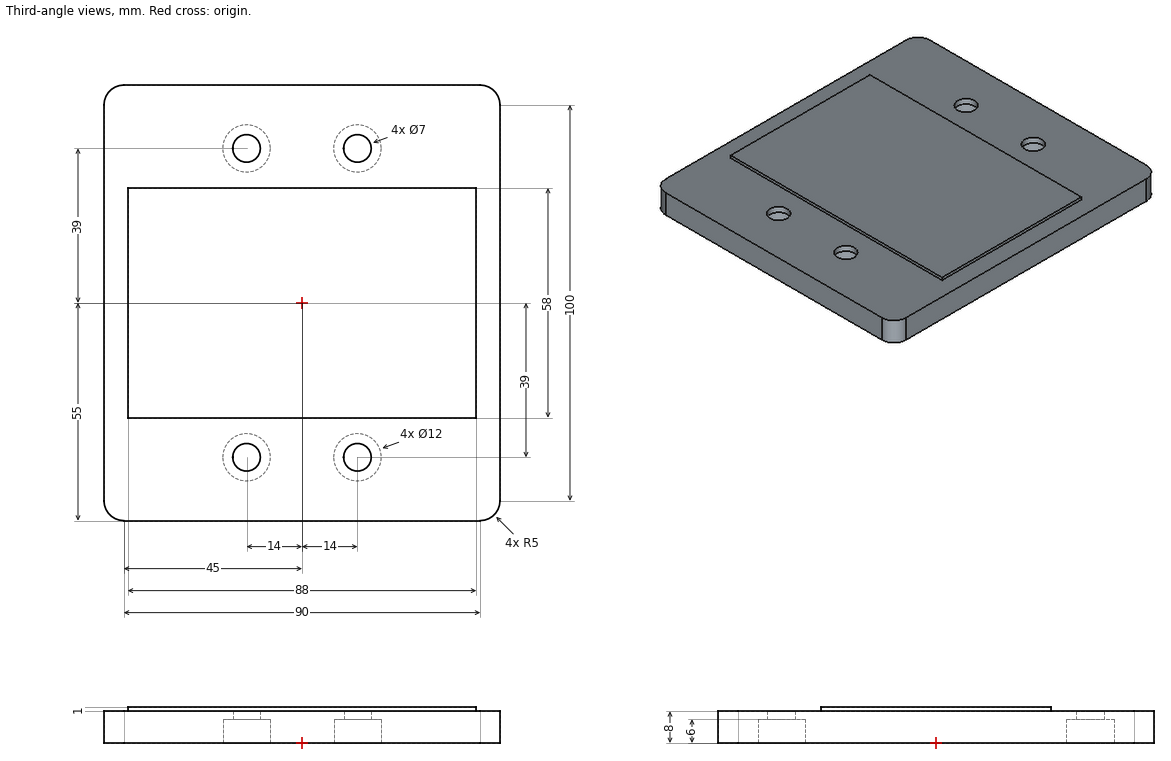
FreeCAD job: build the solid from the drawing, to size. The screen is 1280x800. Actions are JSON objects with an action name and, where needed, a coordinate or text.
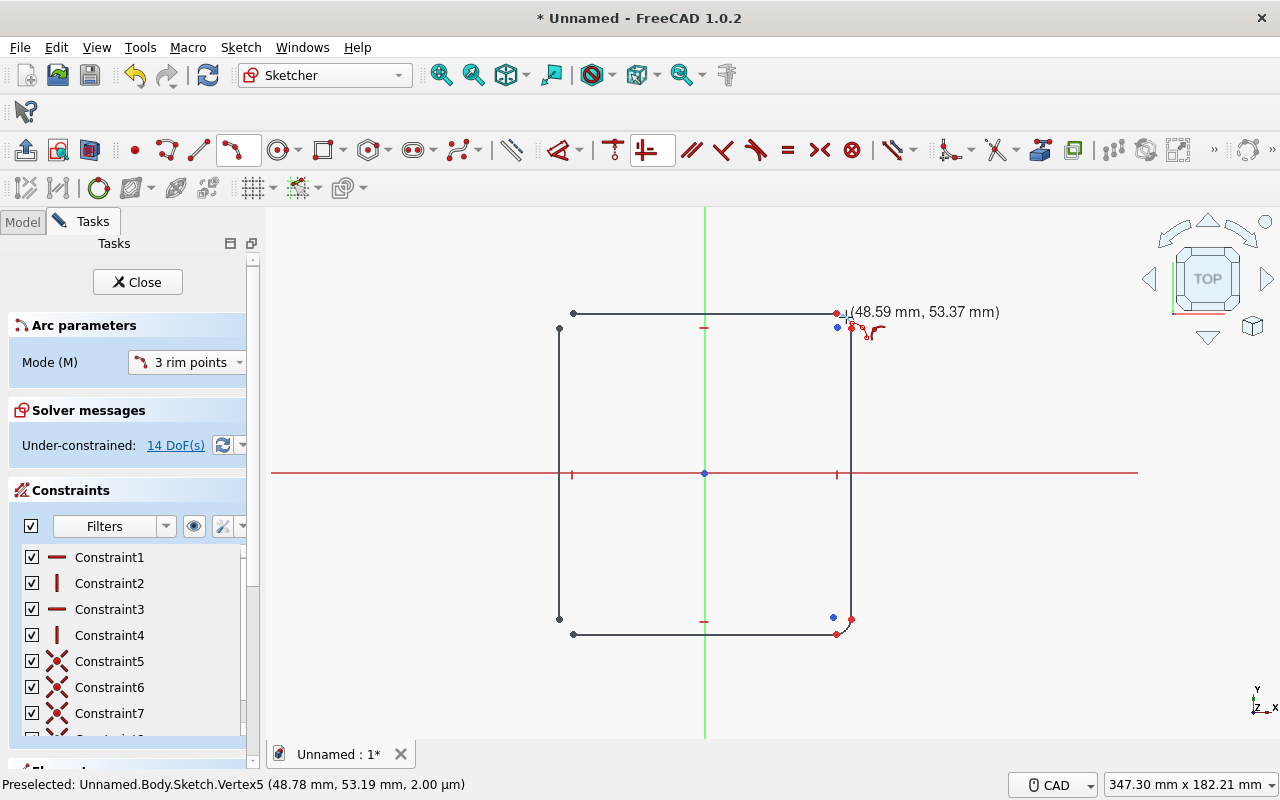
{"action": "left_click", "coordinate": [573, 314]}
{"action": "left_click", "coordinate": [559, 328]}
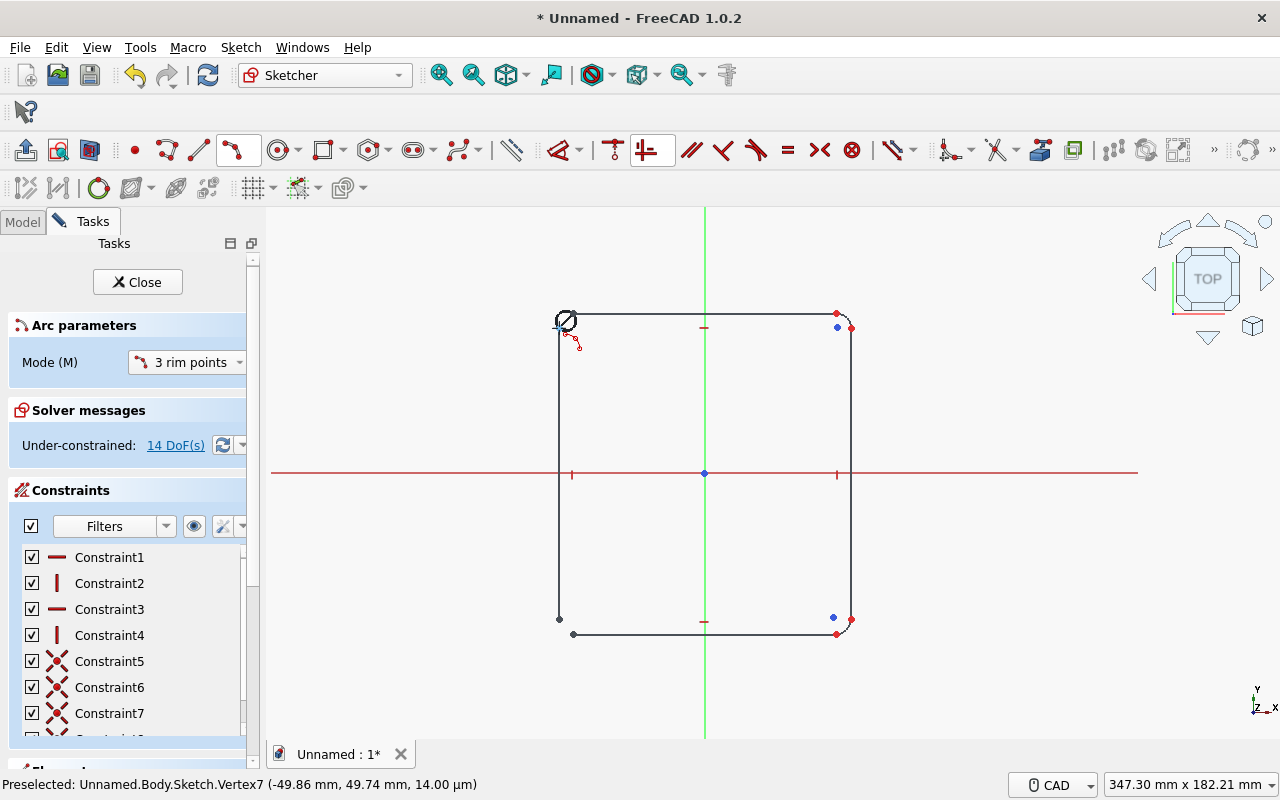
{"action": "scroll", "coordinate": [563, 317], "scroll_direction": "up", "scroll_amount": 7}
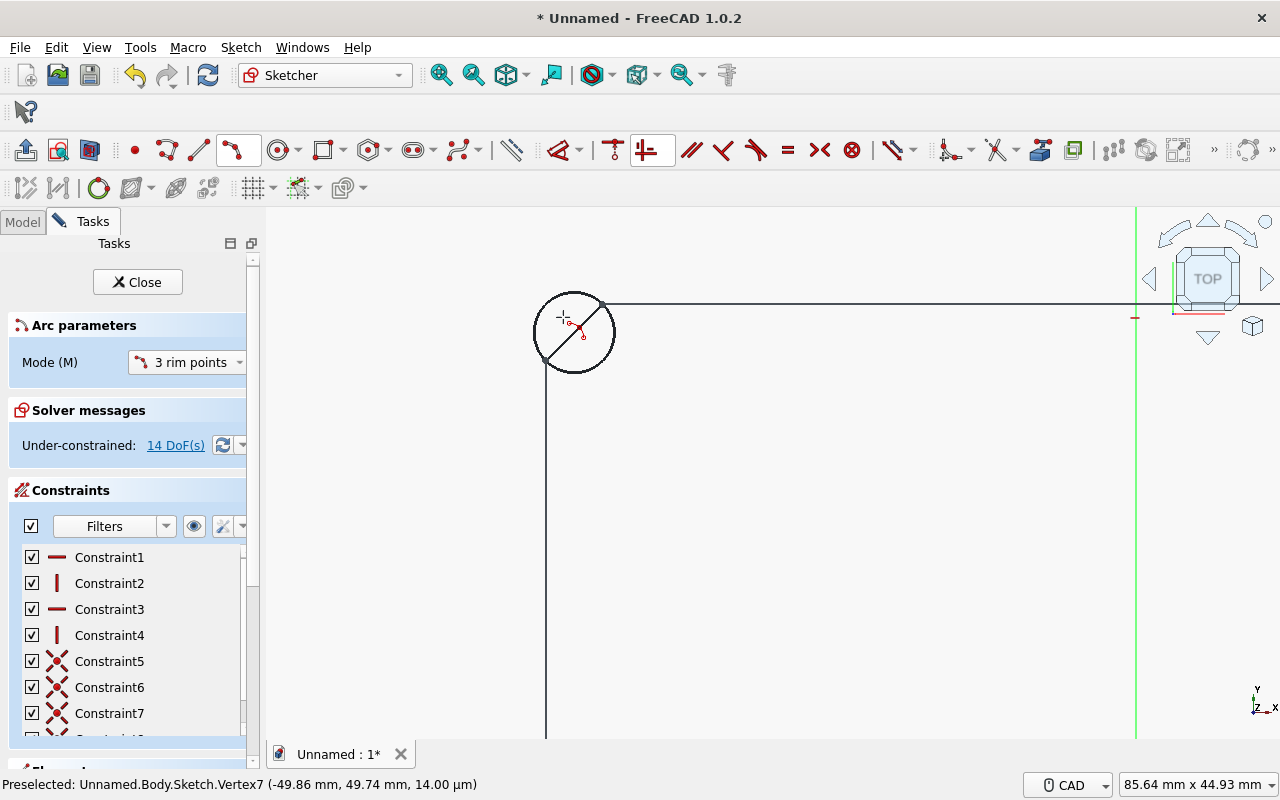
{"action": "left_click", "coordinate": [562, 316]}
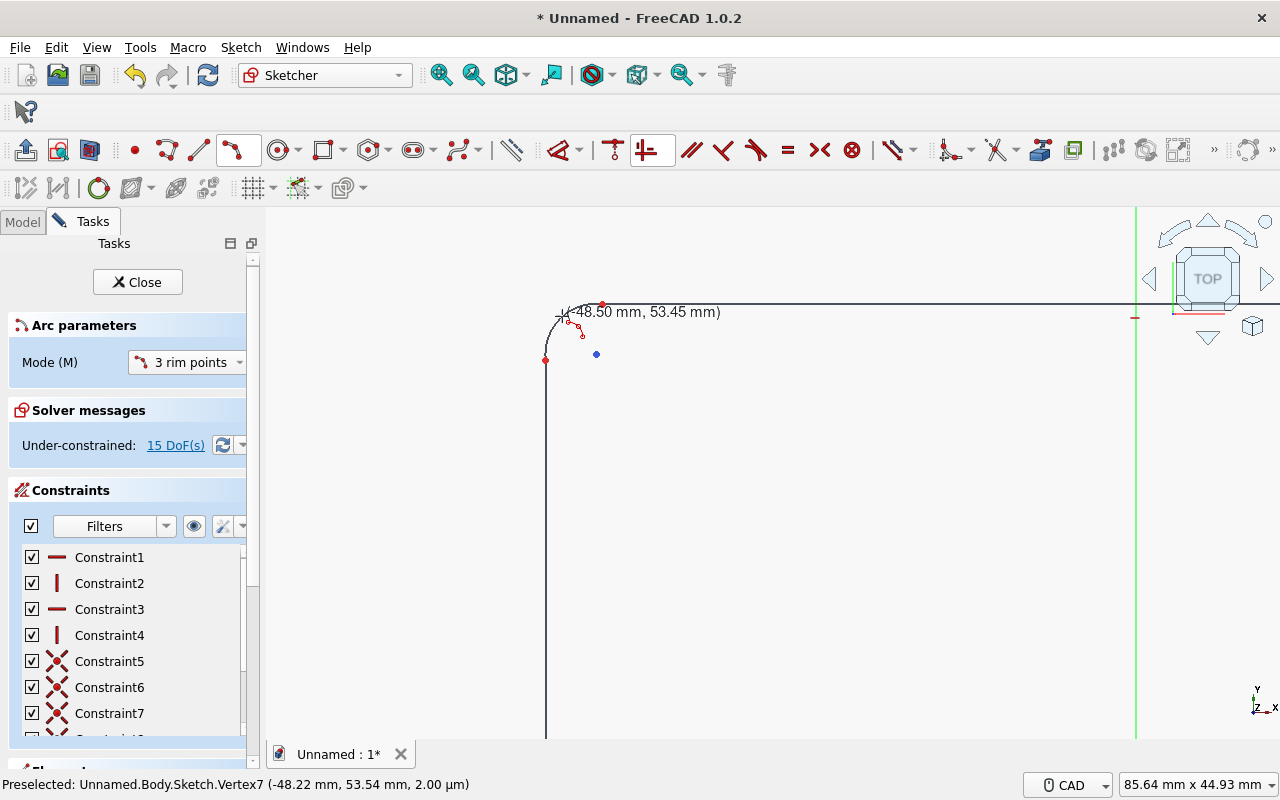
{"action": "scroll", "coordinate": [563, 317], "scroll_direction": "down", "scroll_amount": 7}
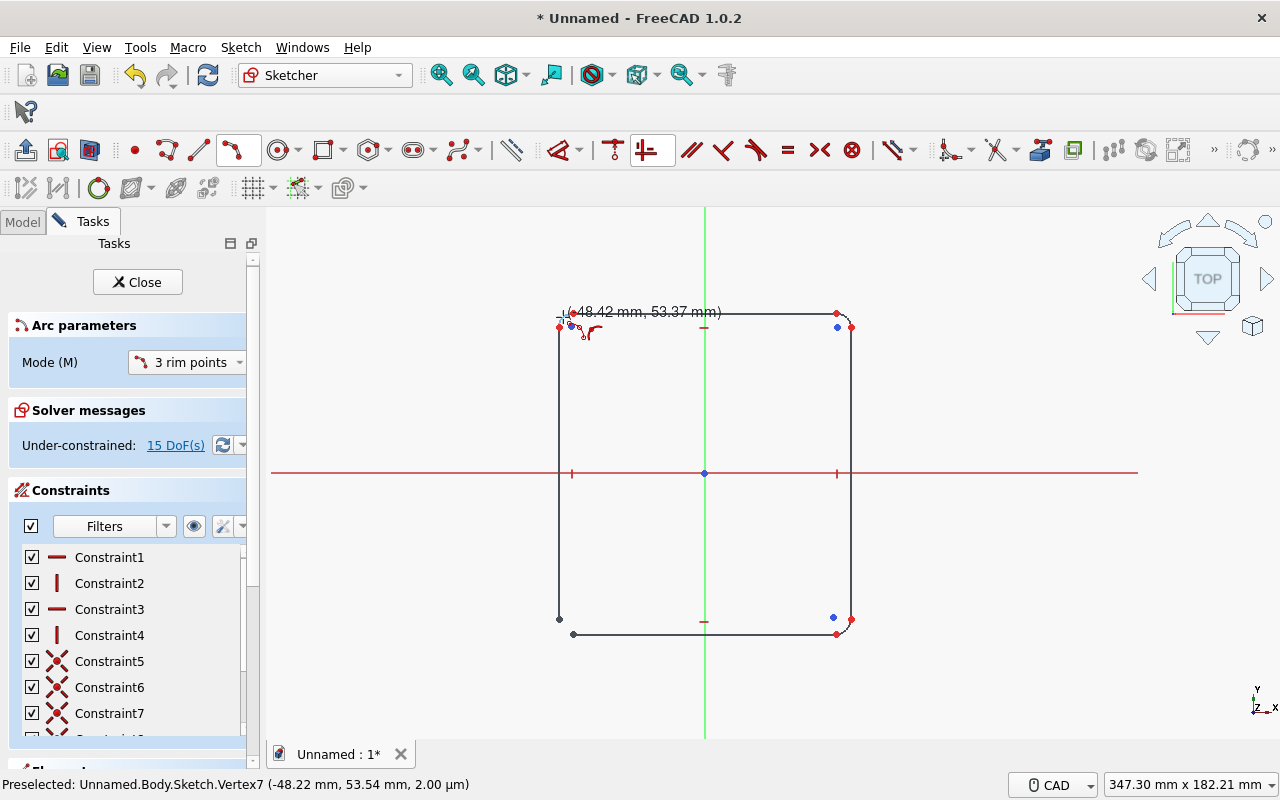
{"action": "left_click", "coordinate": [559, 620]}
{"action": "left_click", "coordinate": [573, 635]}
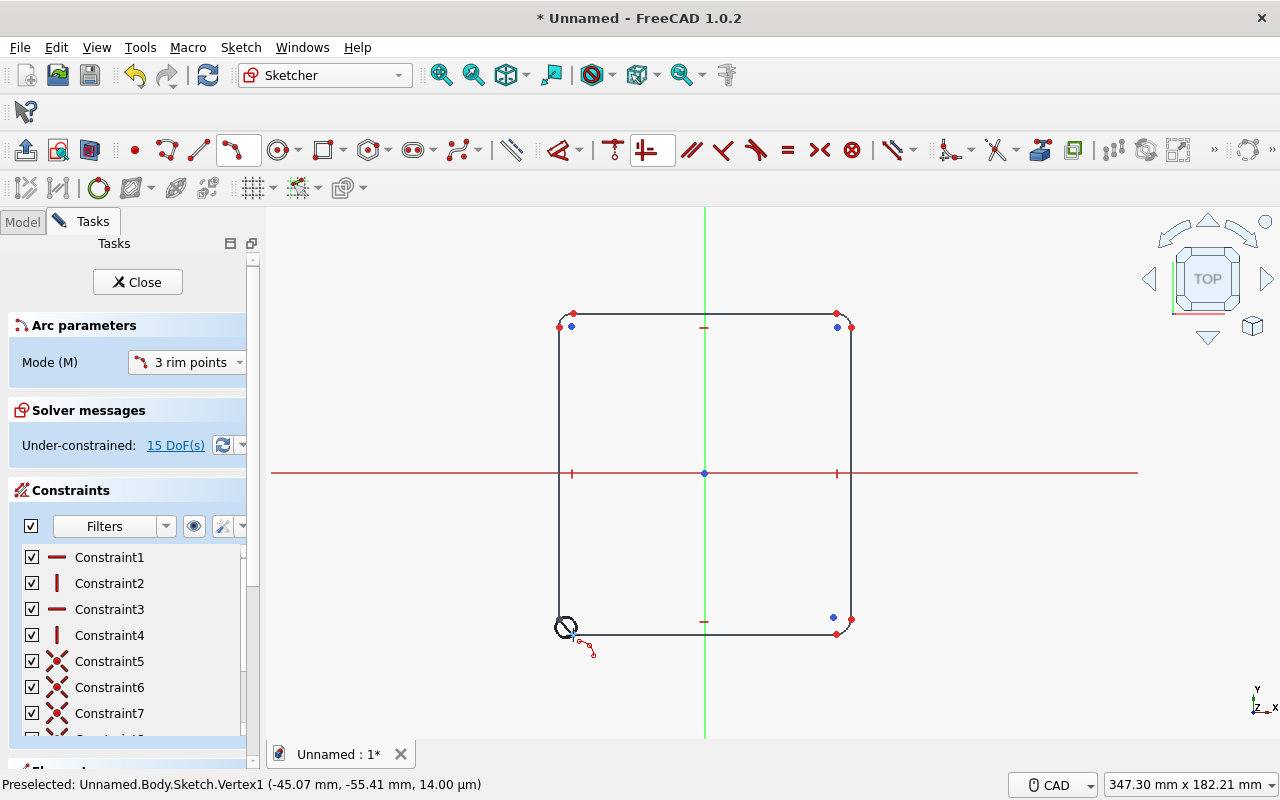
{"action": "scroll", "coordinate": [563, 630], "scroll_direction": "up", "scroll_amount": 7}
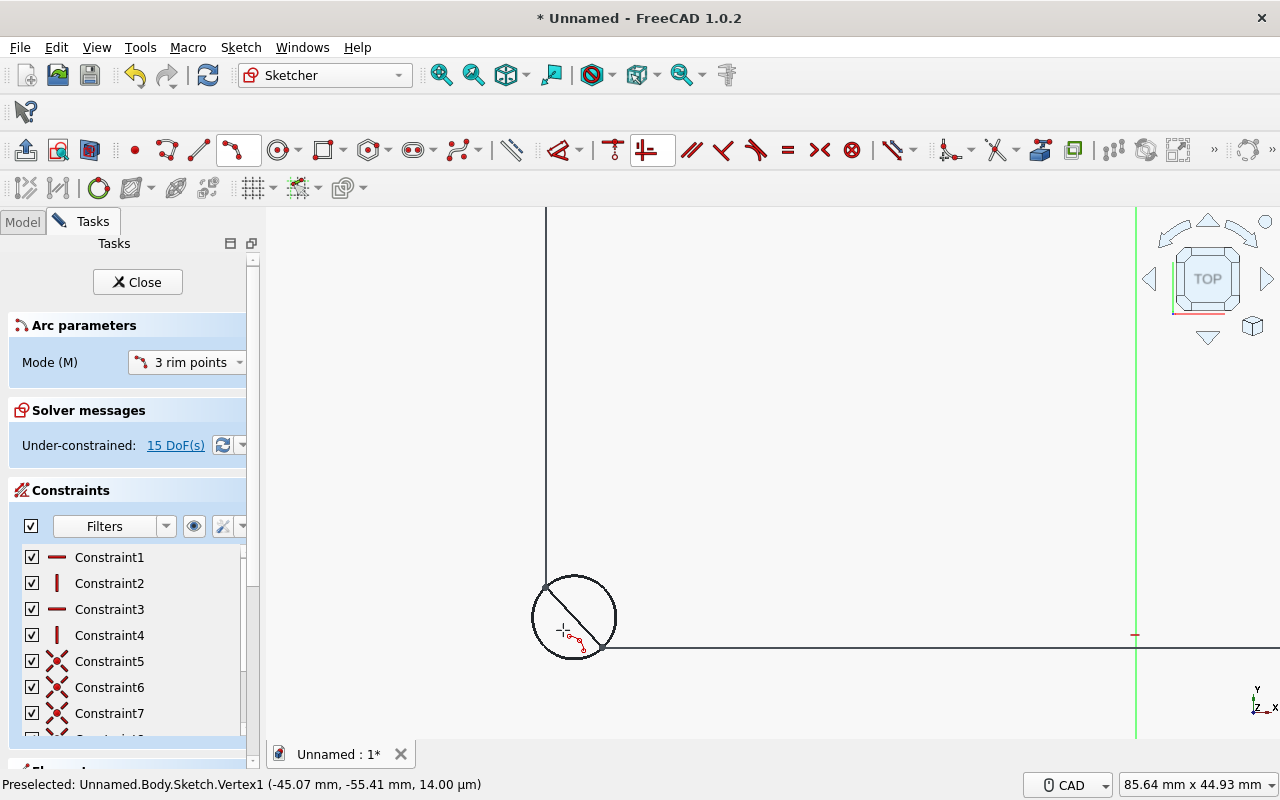
{"action": "left_click", "coordinate": [562, 626]}
{"action": "key", "text": "Escape"}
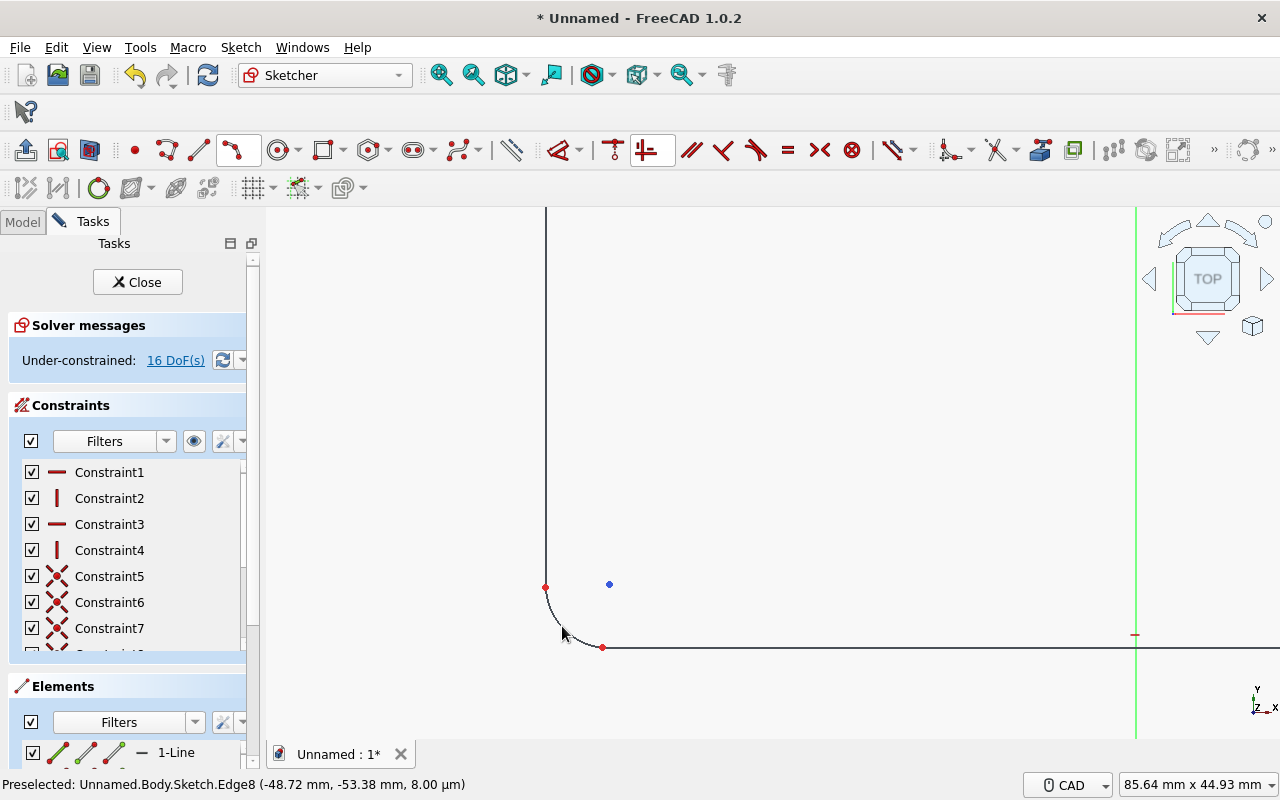
{"action": "scroll", "coordinate": [563, 630], "scroll_direction": "down", "scroll_amount": 7}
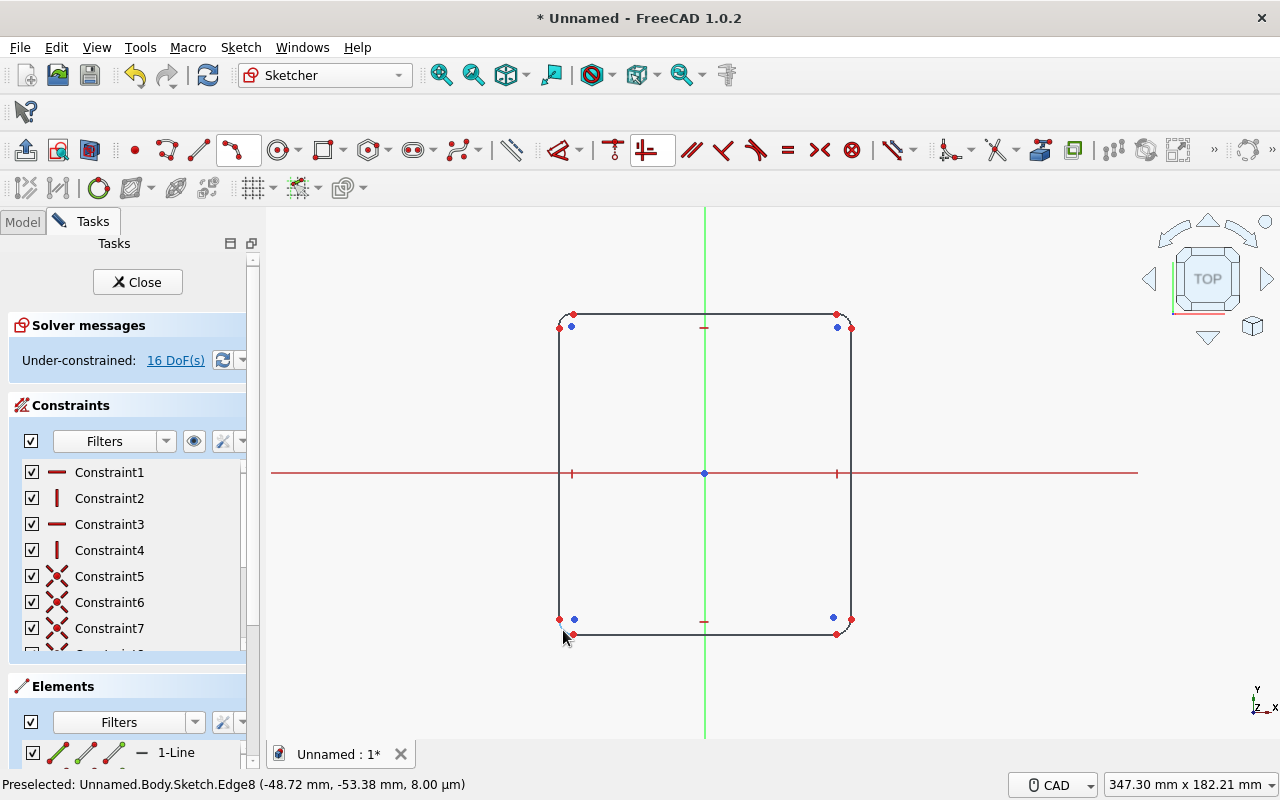
{"action": "left_click", "coordinate": [652, 635]}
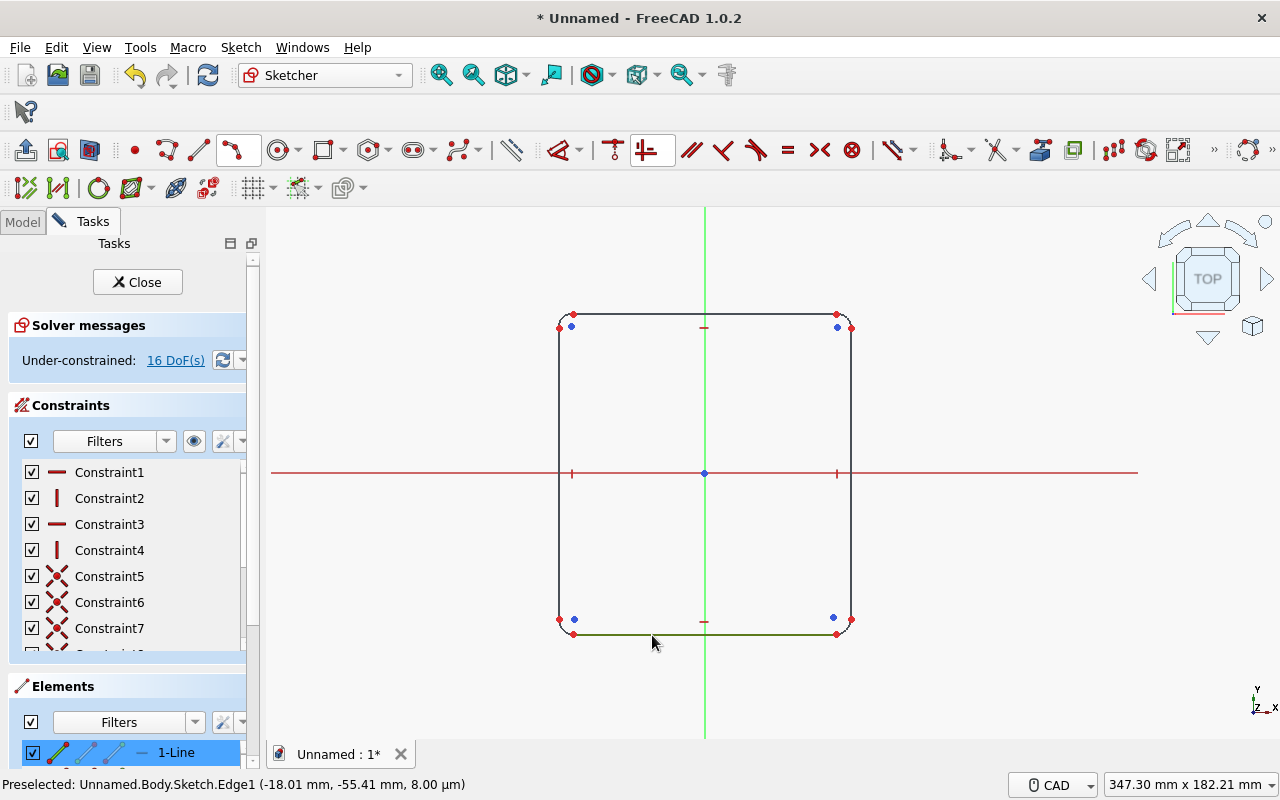
{"action": "scroll", "coordinate": [846, 630], "scroll_direction": "up", "scroll_amount": 2}